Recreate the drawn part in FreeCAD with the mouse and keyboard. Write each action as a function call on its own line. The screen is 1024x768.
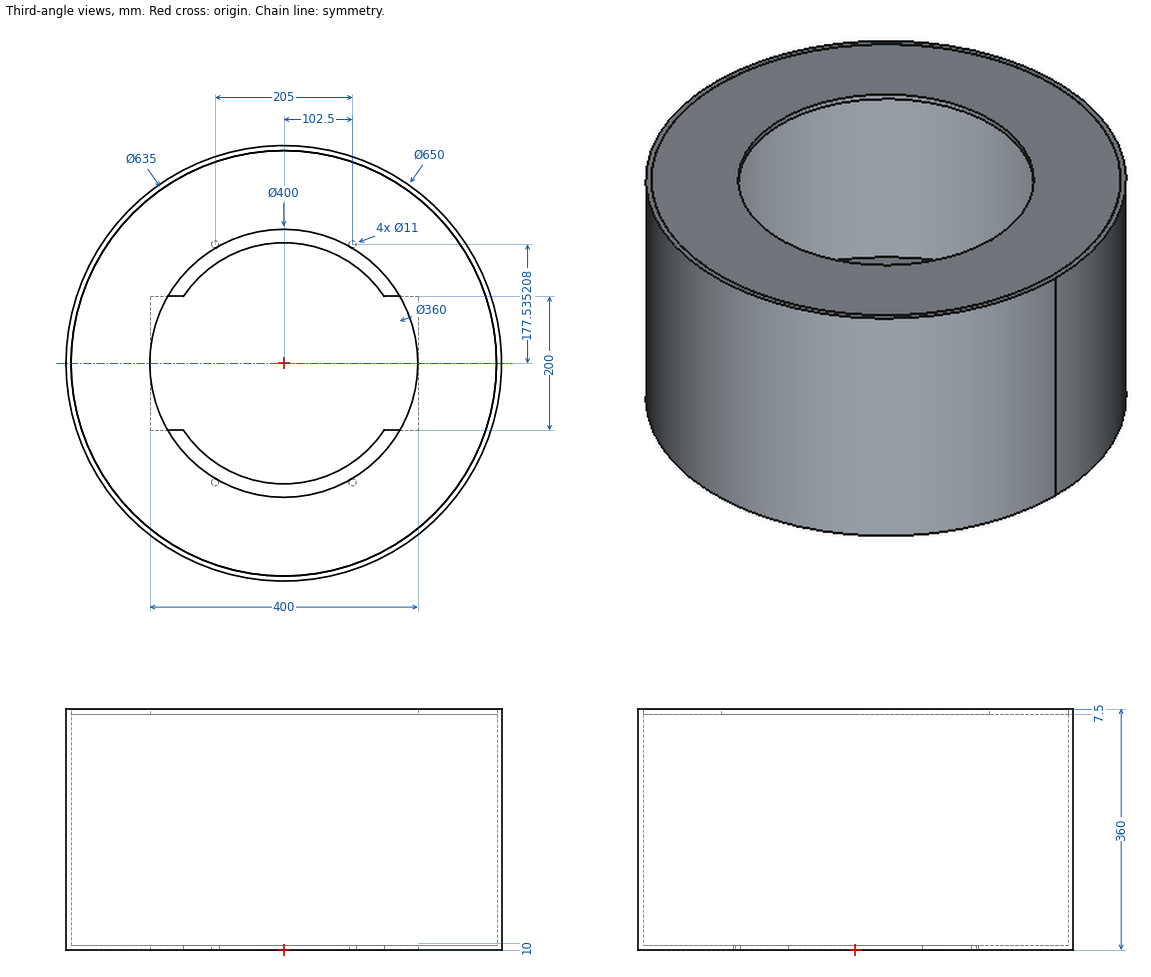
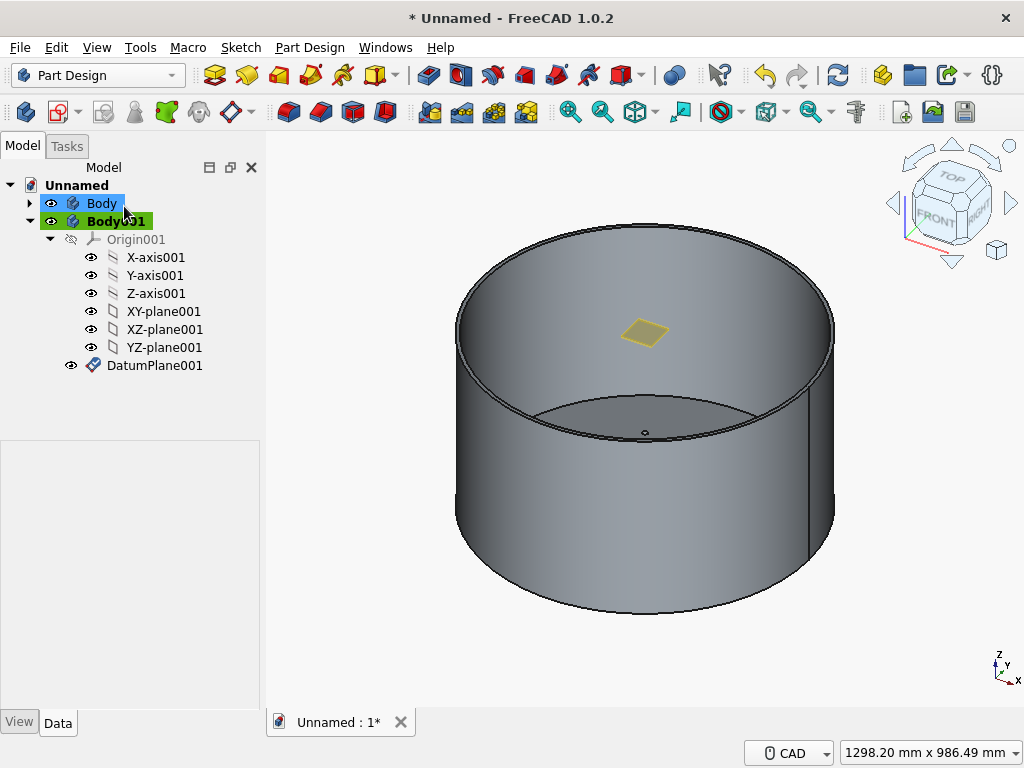
click(116, 365)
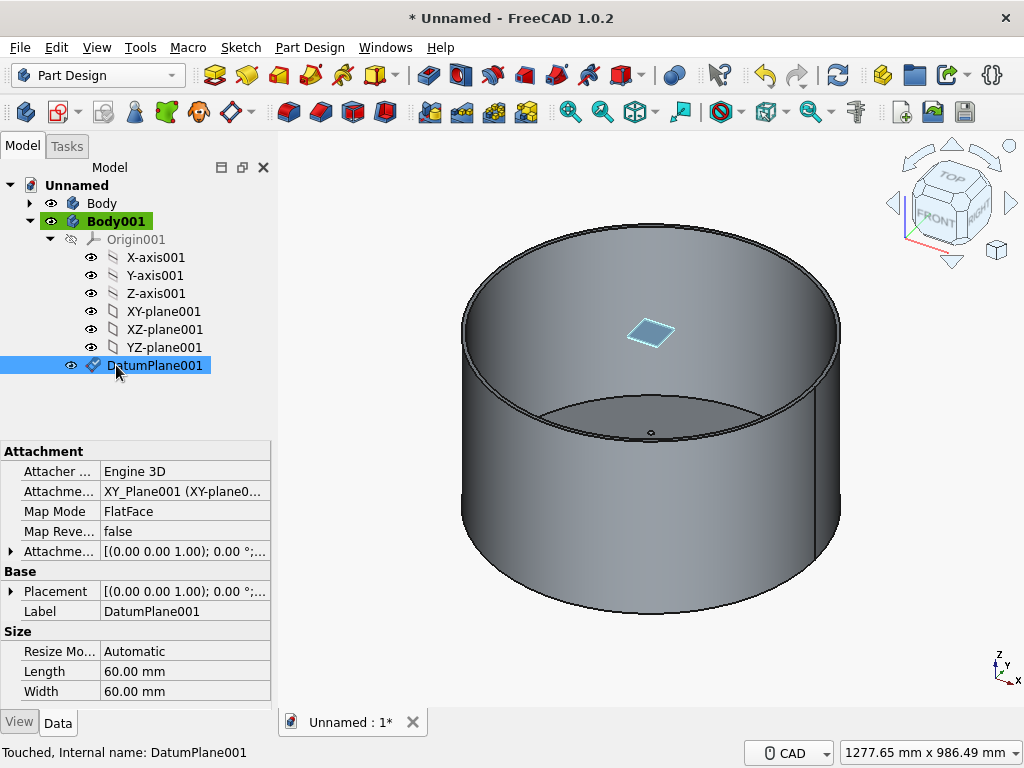
click(58, 112)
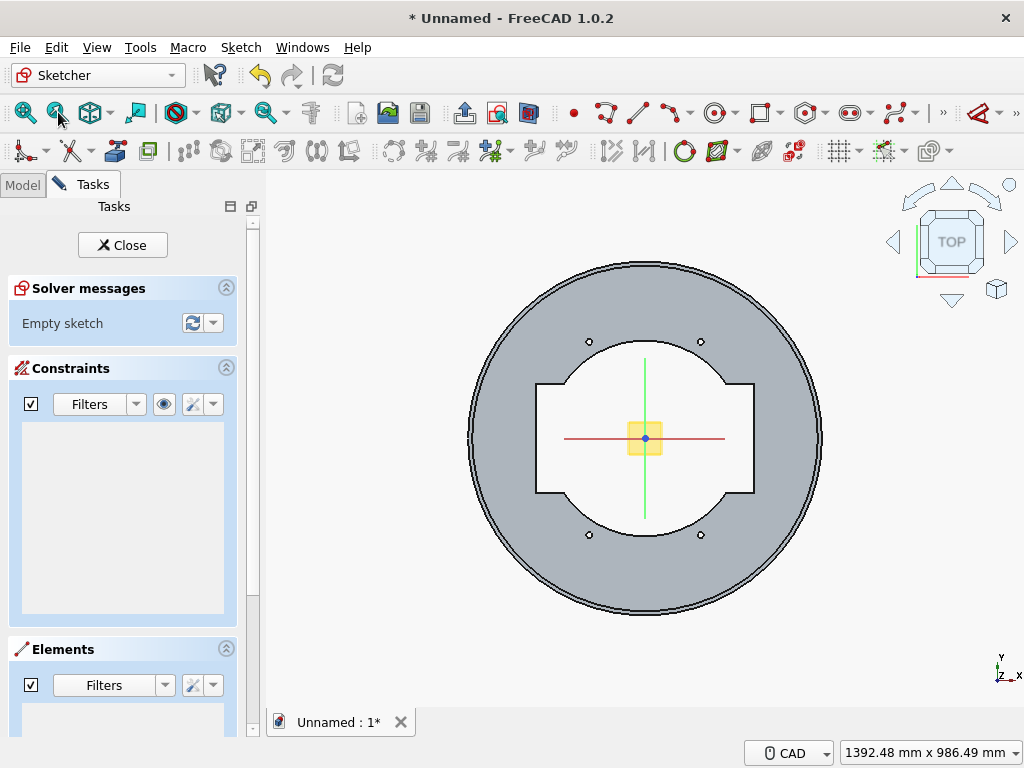
click(716, 114)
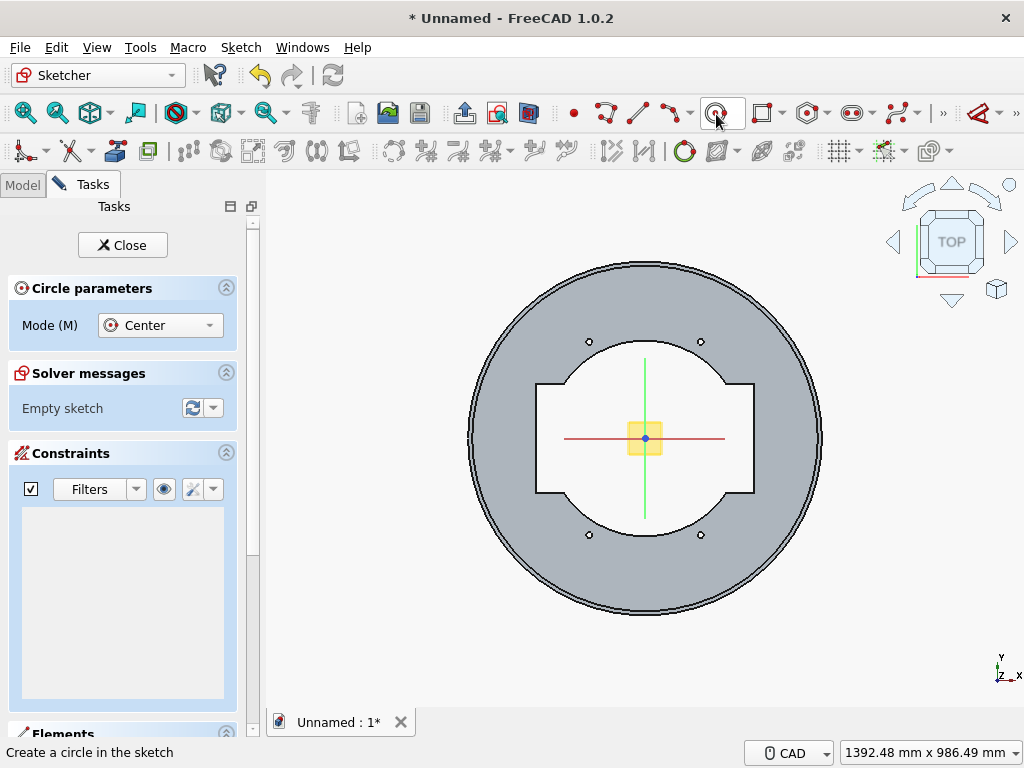
click(645, 438)
click(767, 316)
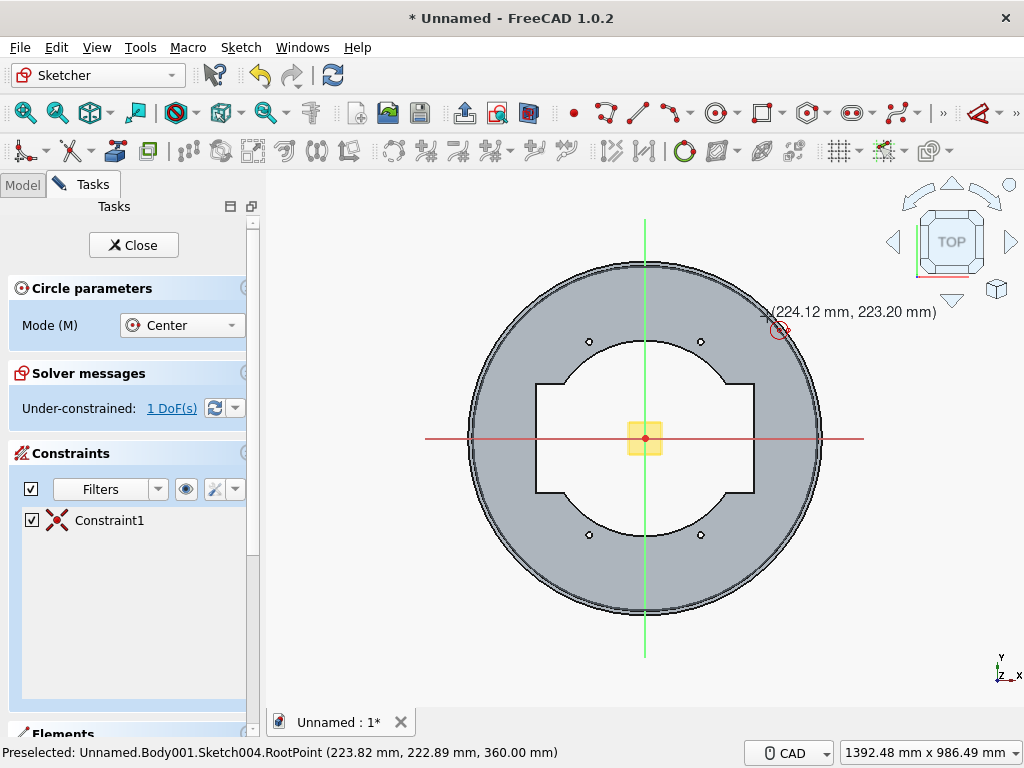
click(645, 438)
click(722, 362)
key(Escape)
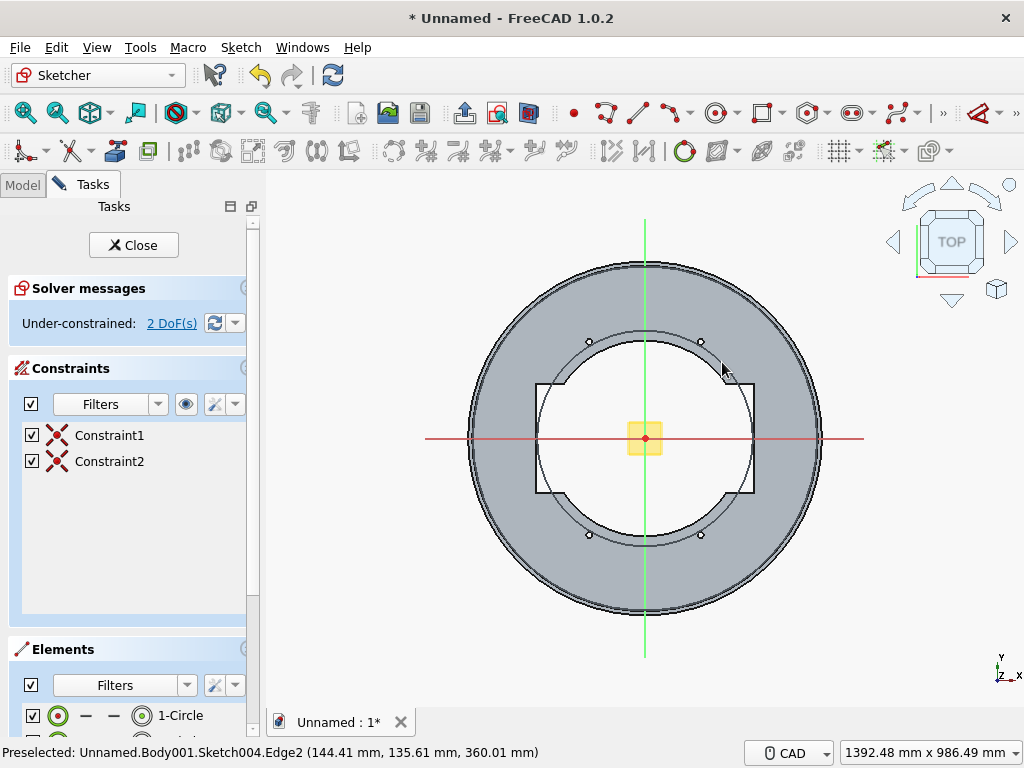
click(978, 114)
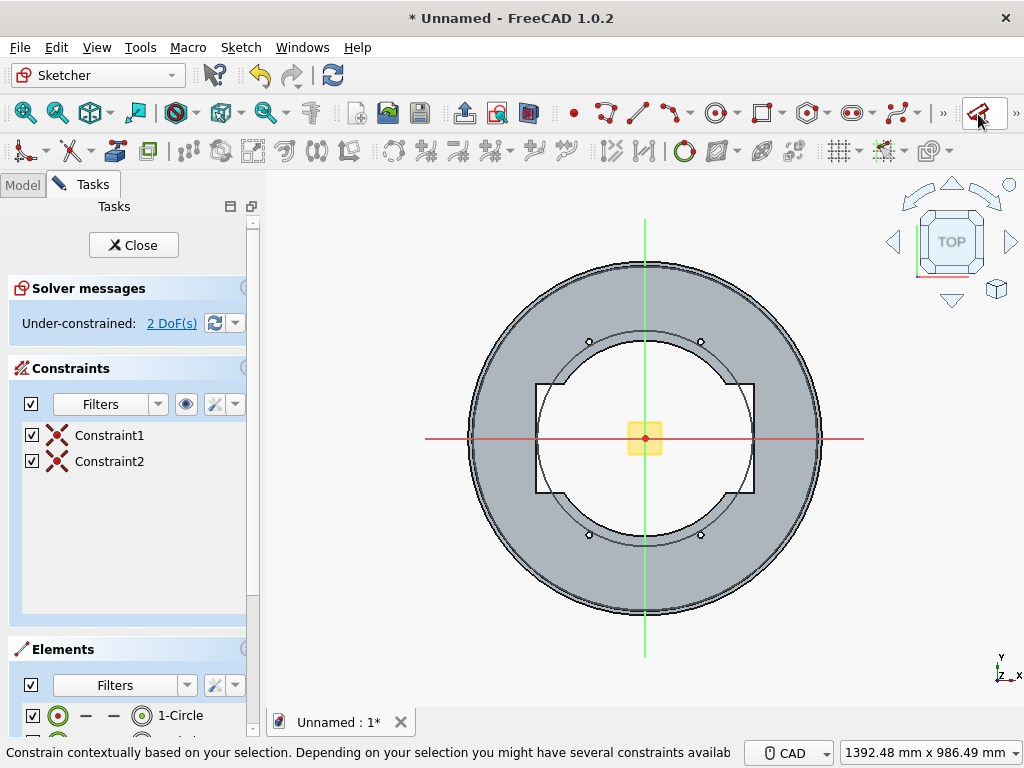
click(766, 316)
click(788, 293)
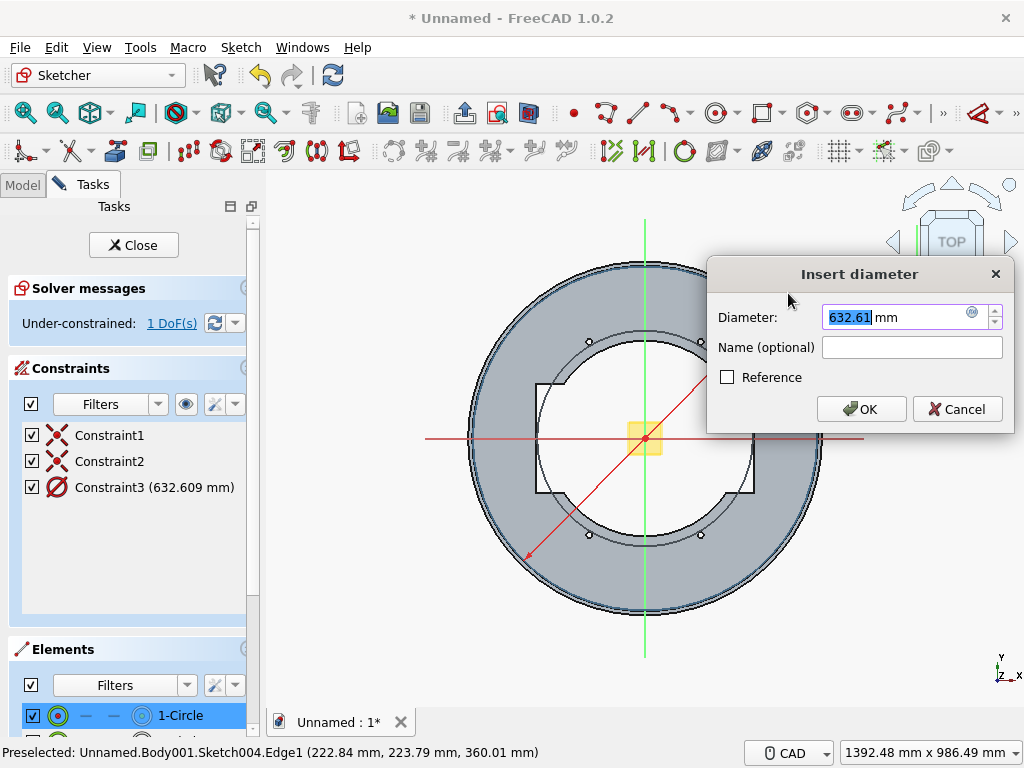
text(635)
key(Return)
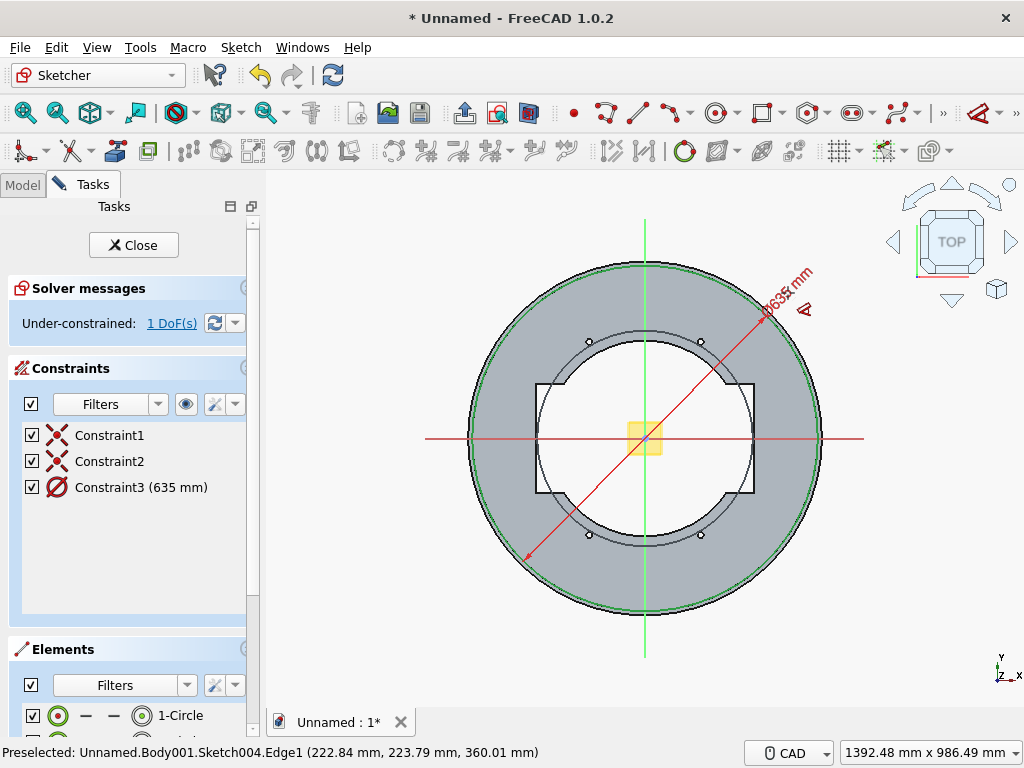
click(721, 362)
click(744, 339)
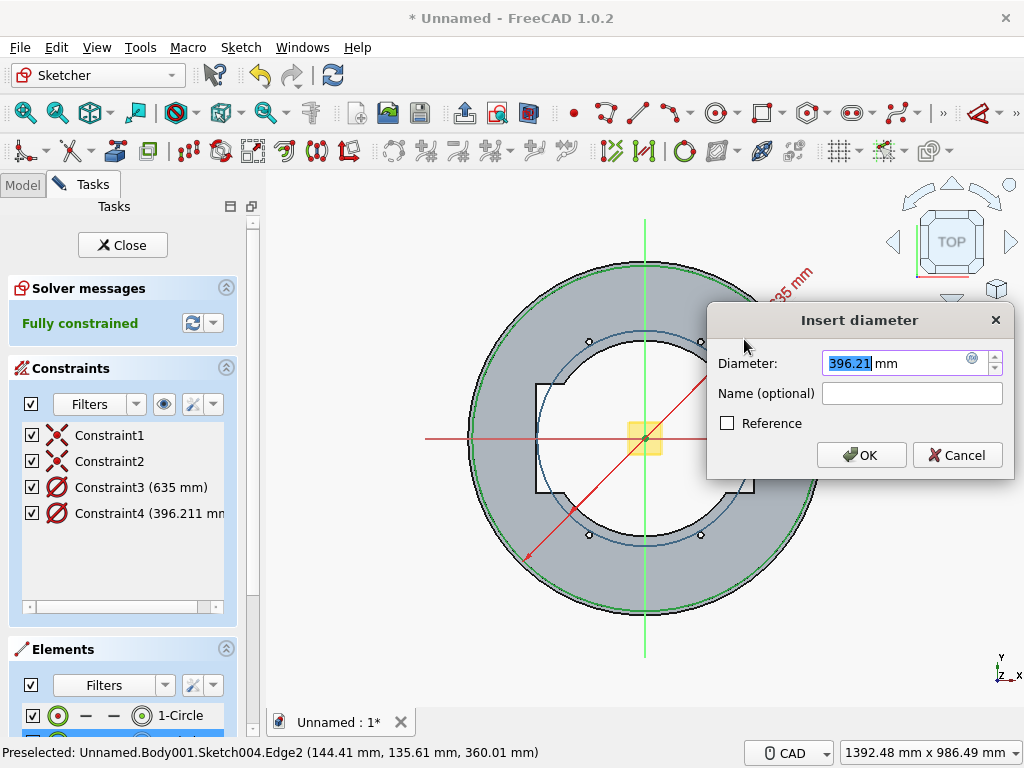
text(400)
key(Return)
key(Escape)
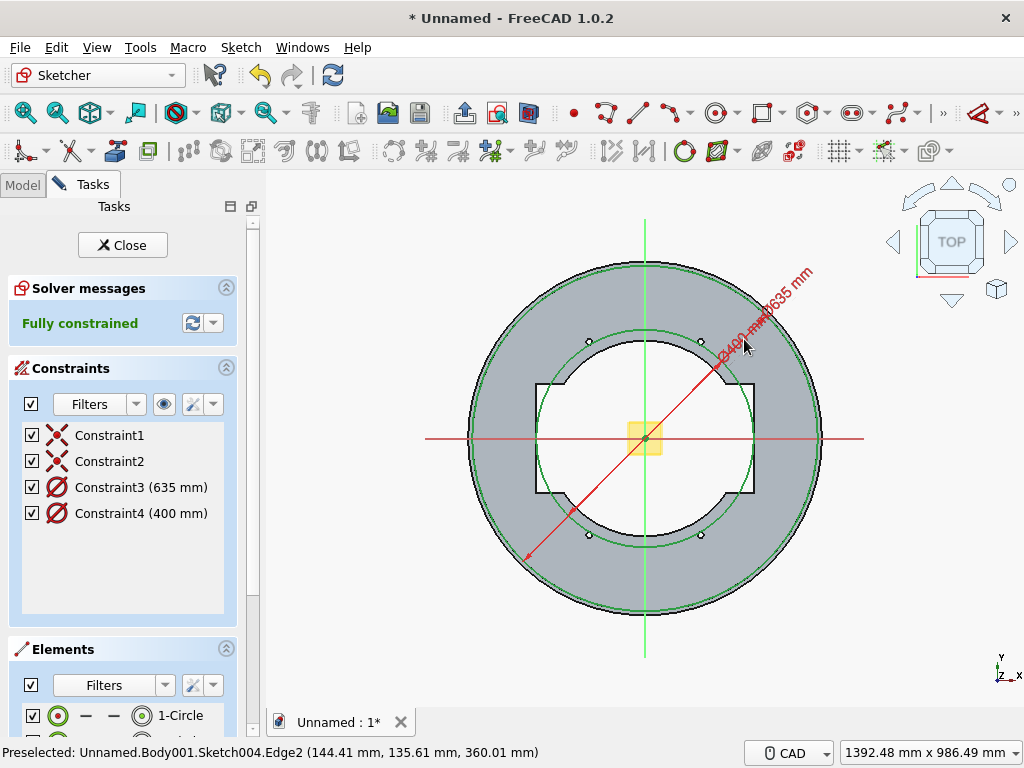
click(123, 245)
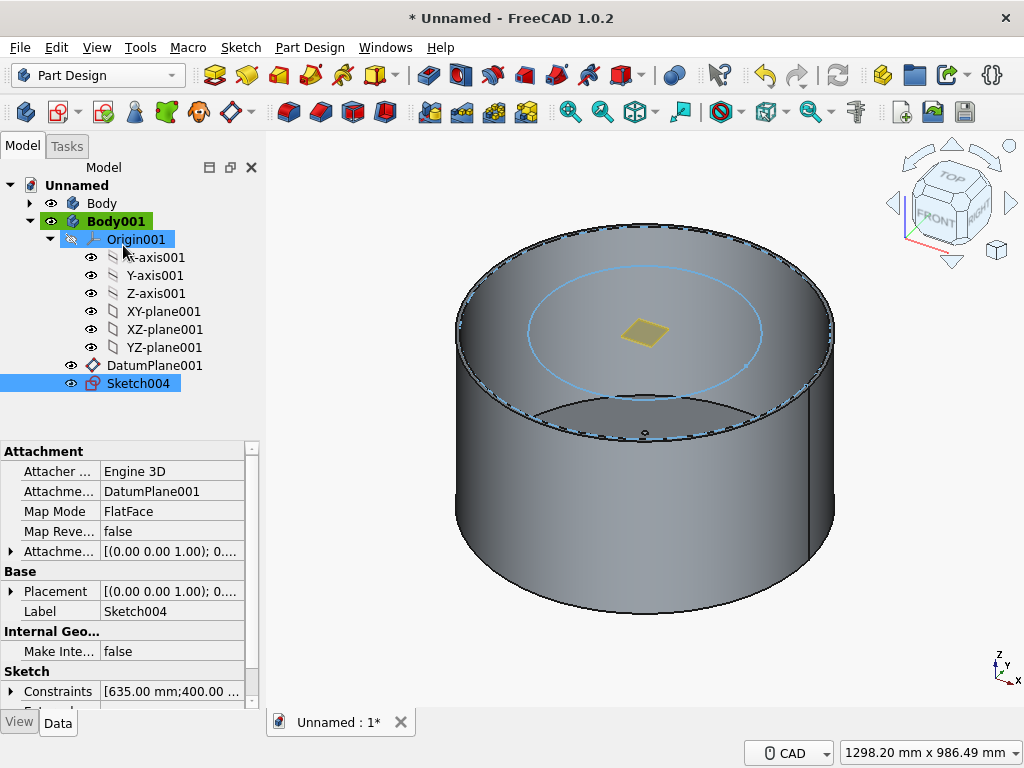
click(216, 76)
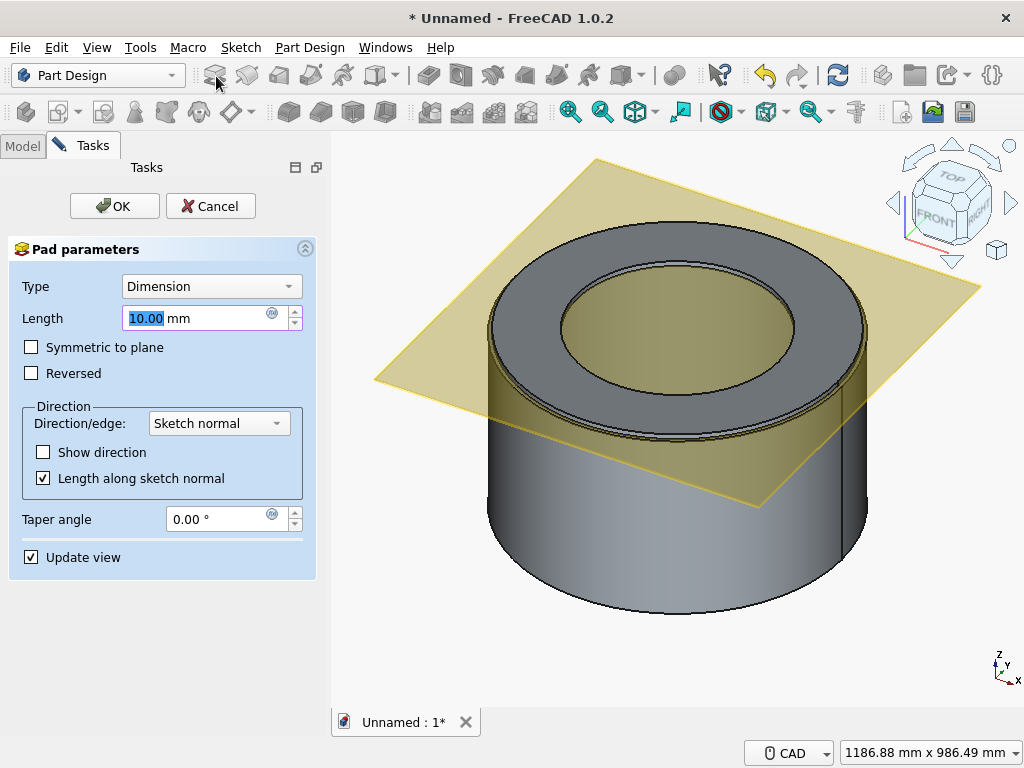
text(7.5)
key(Tab)